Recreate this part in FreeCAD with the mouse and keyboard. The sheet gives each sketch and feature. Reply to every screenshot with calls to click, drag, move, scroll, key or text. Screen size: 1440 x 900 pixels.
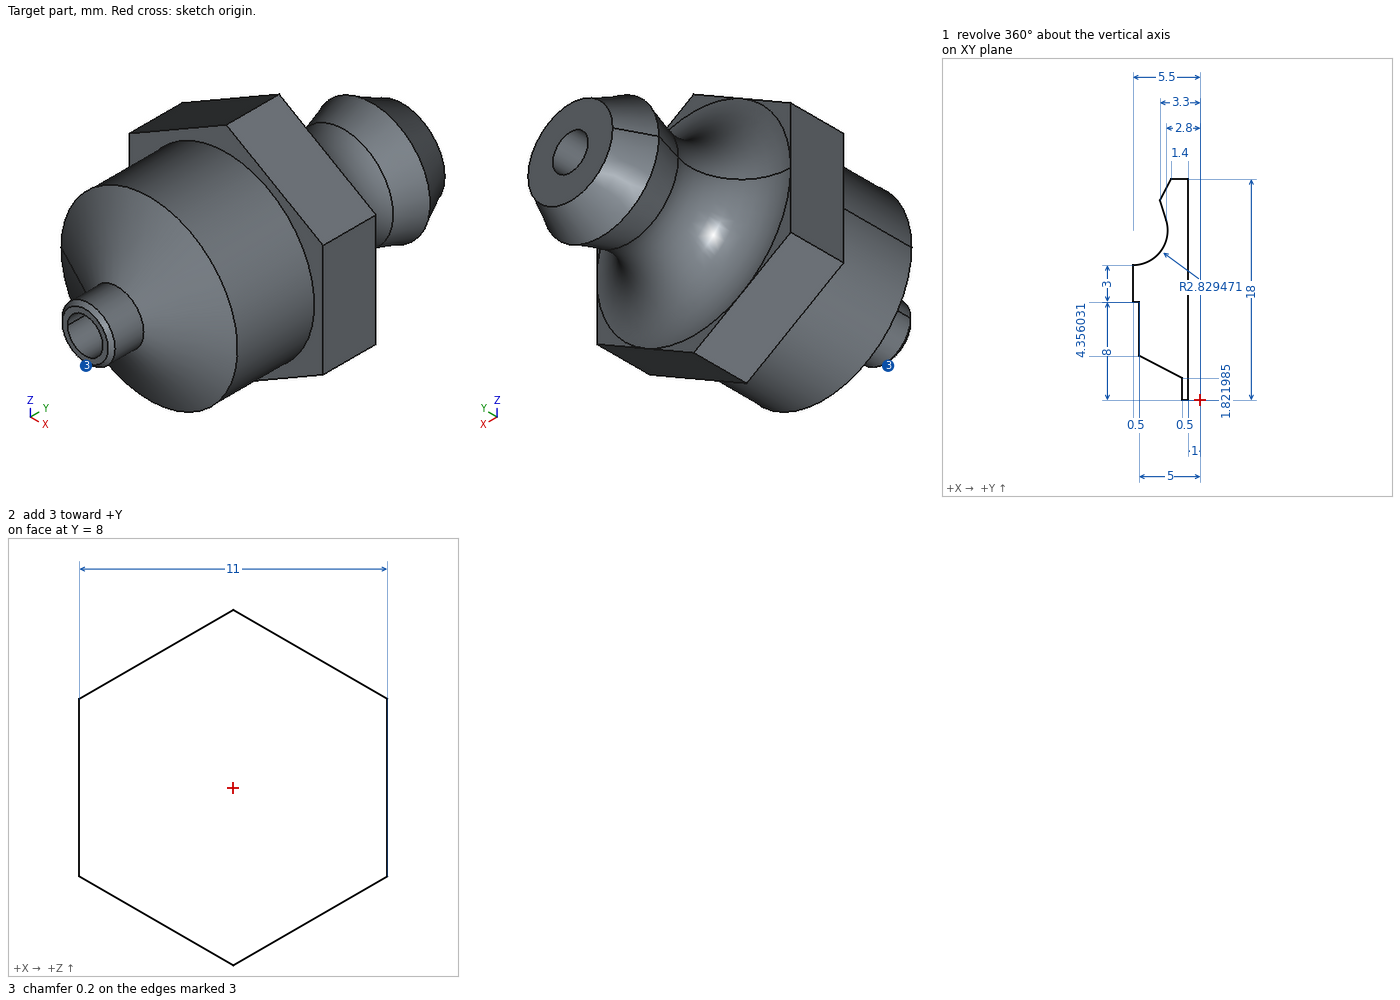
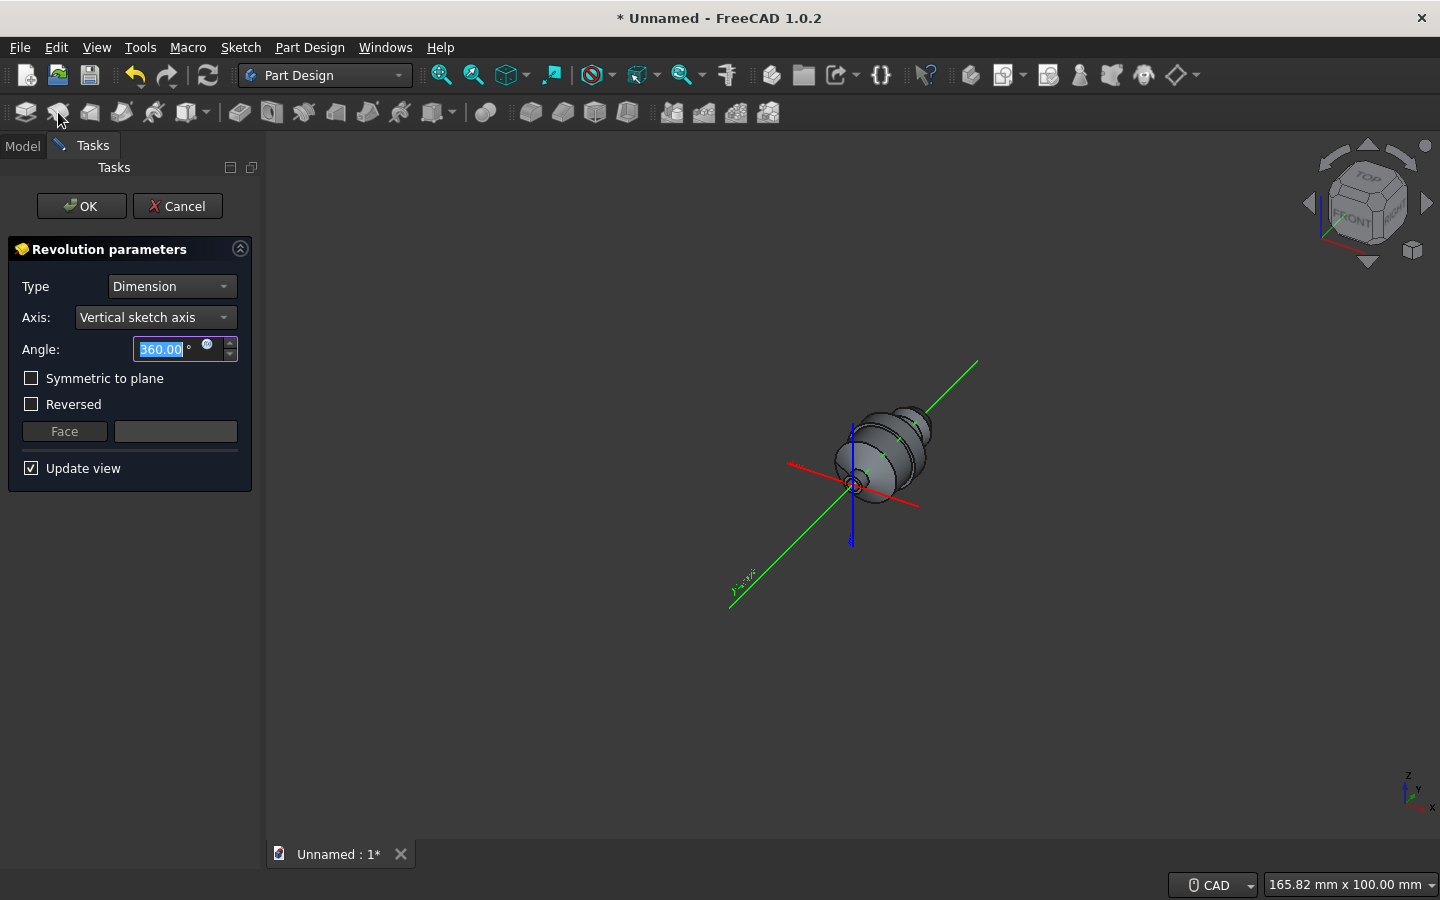
click(82, 206)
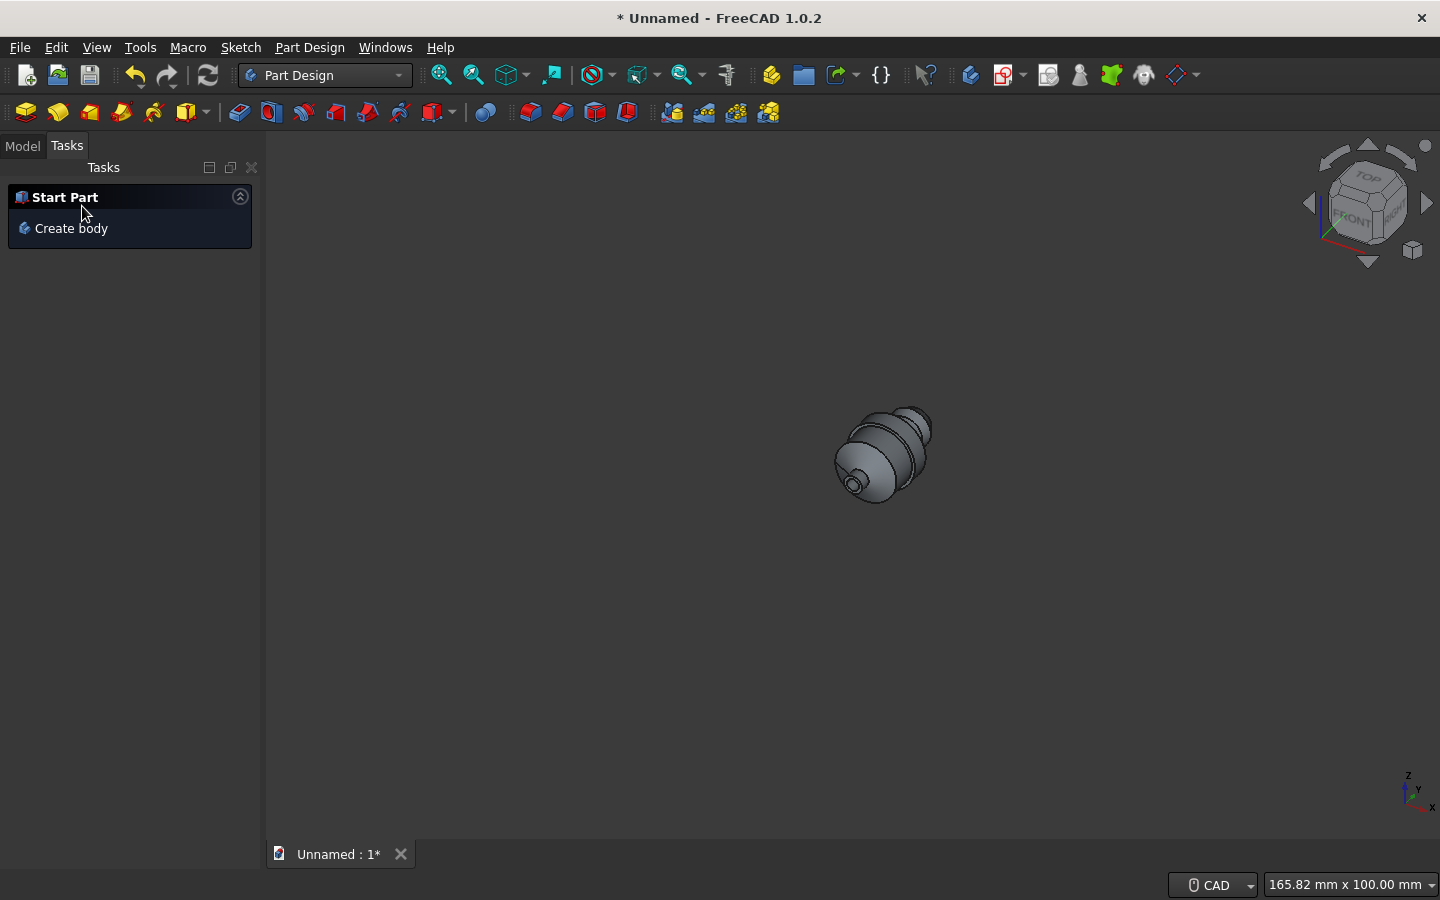
click(442, 76)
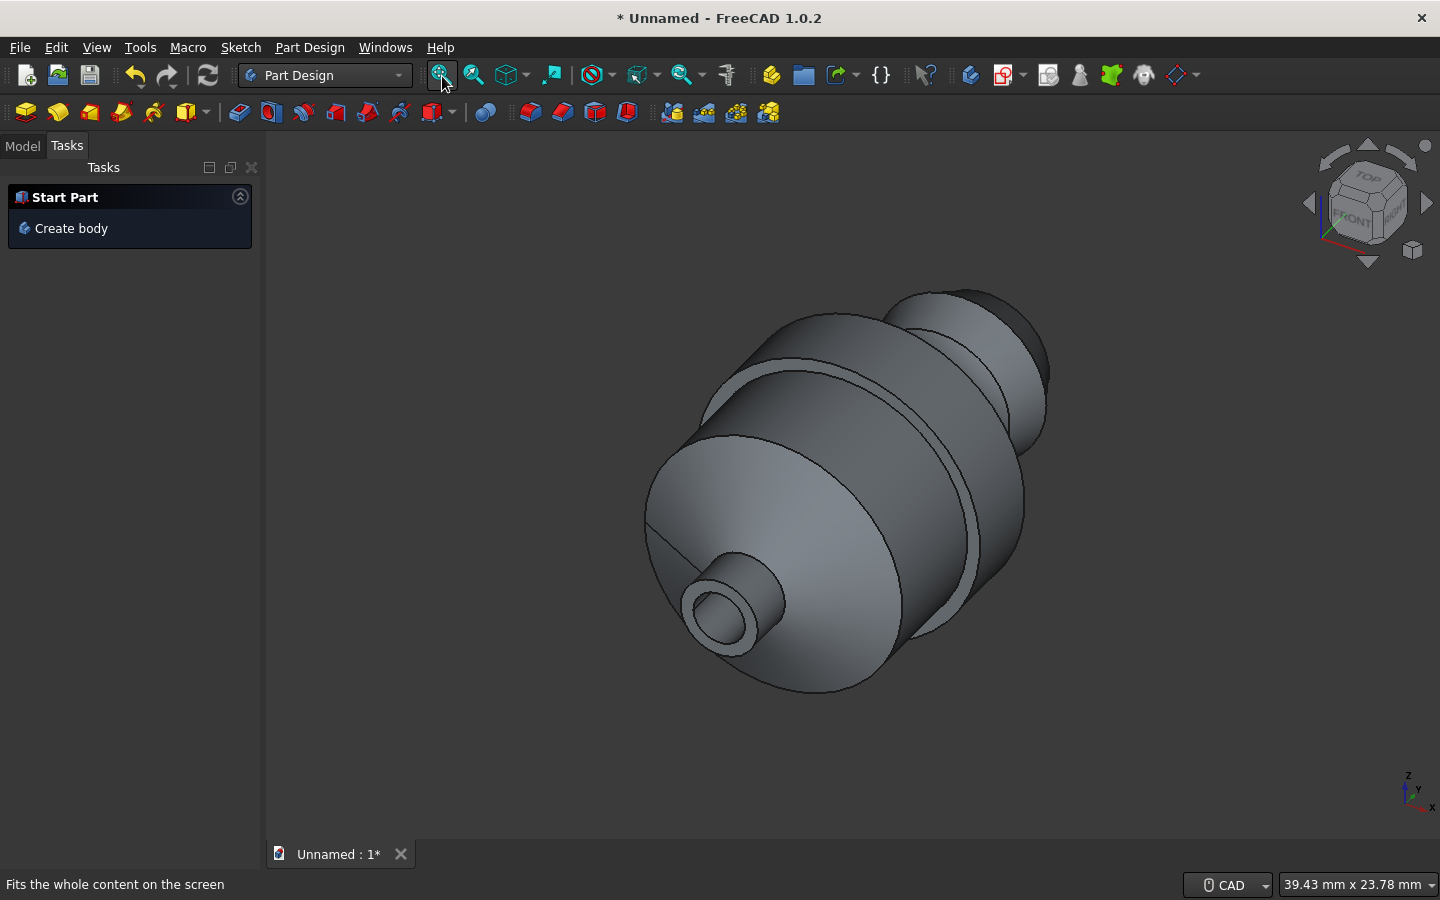
scroll(976, 542, up, 5)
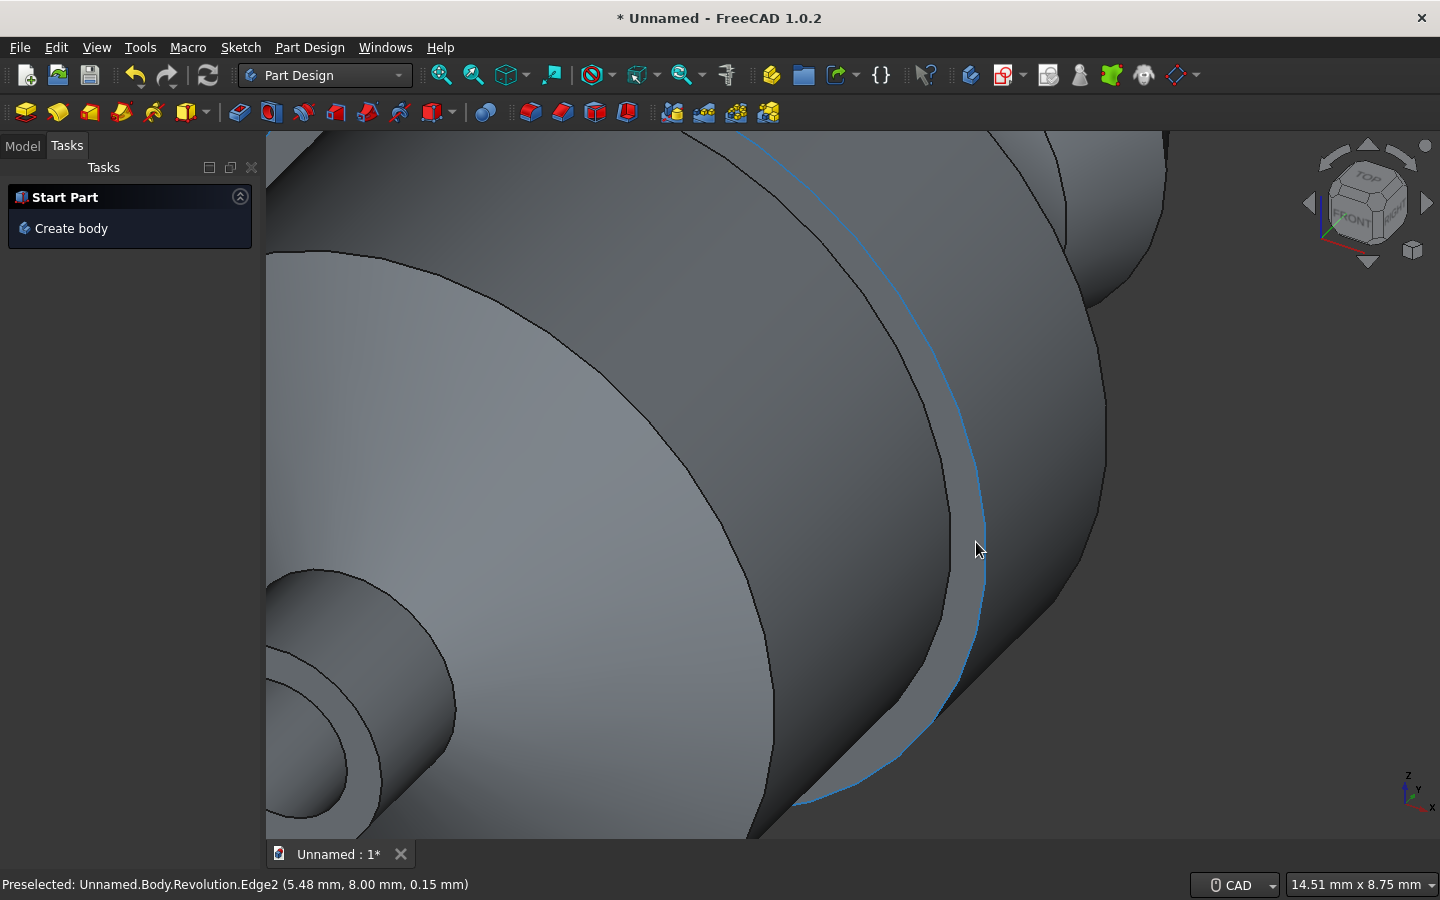
click(974, 543)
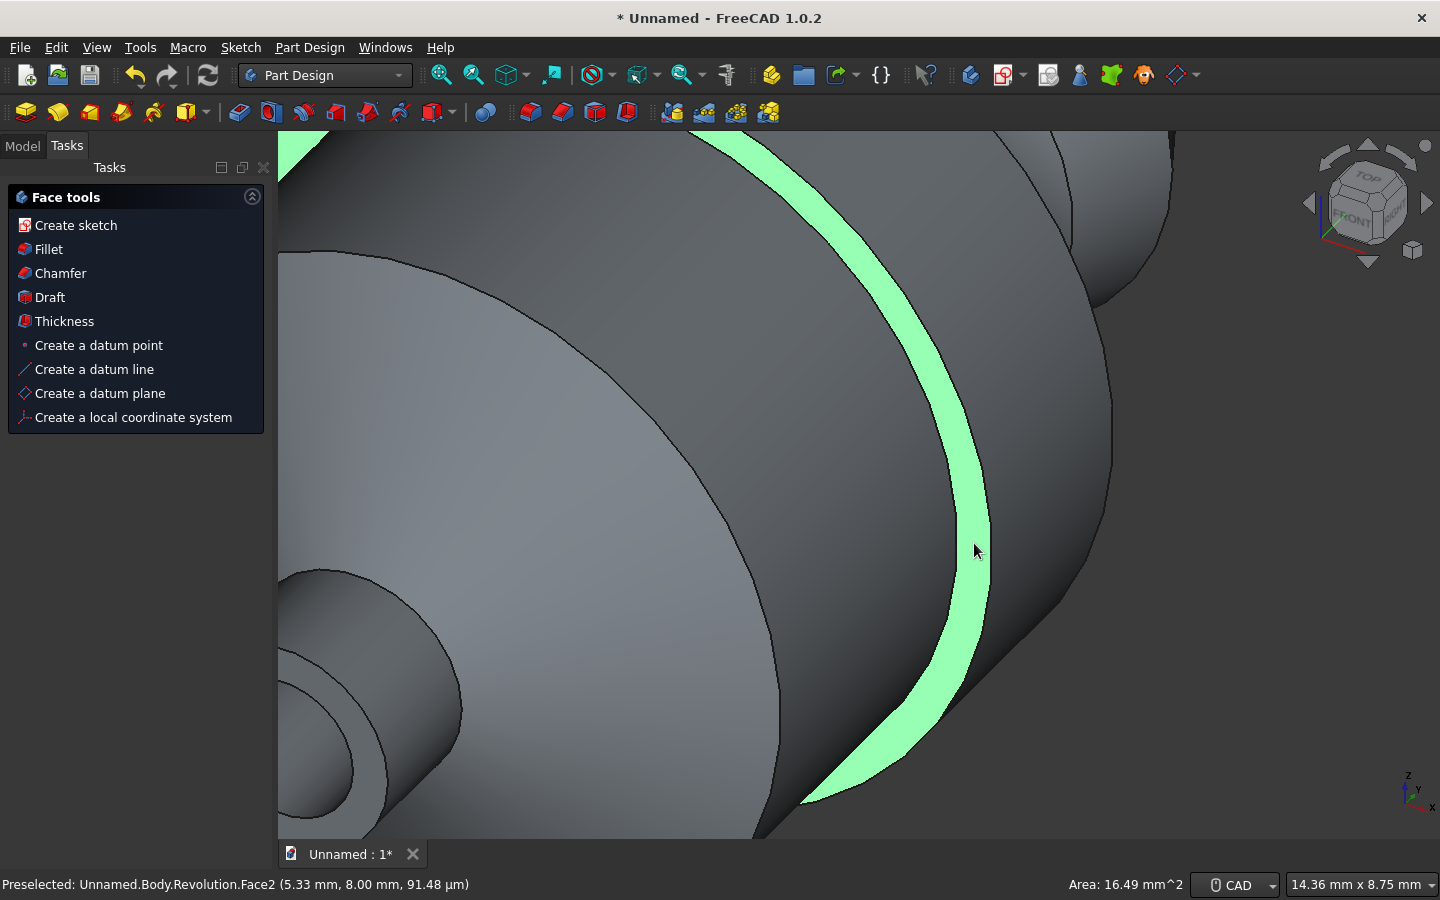
click(1004, 76)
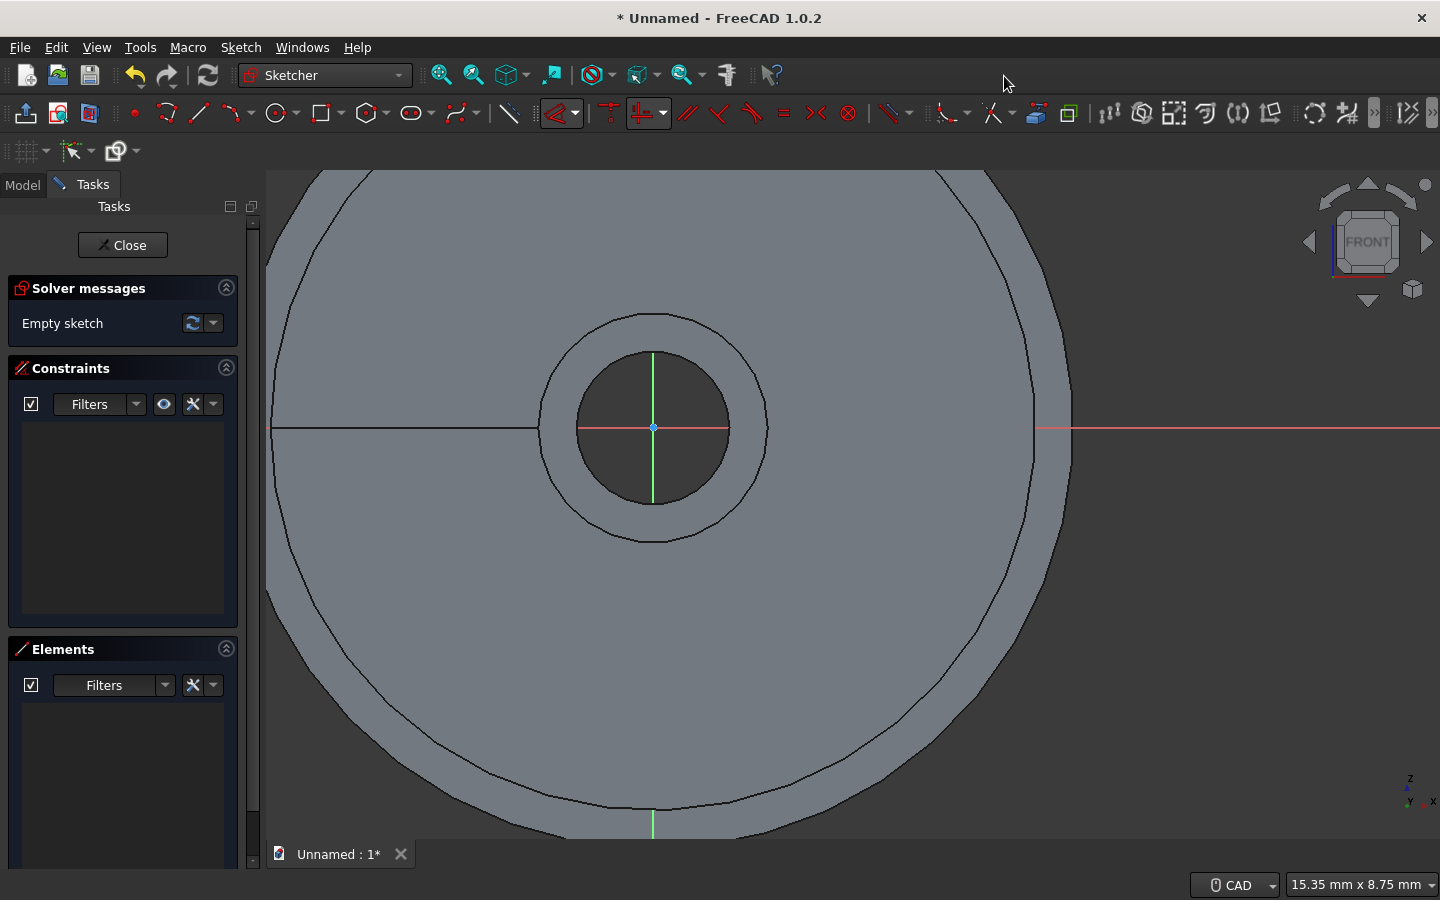
click(90, 114)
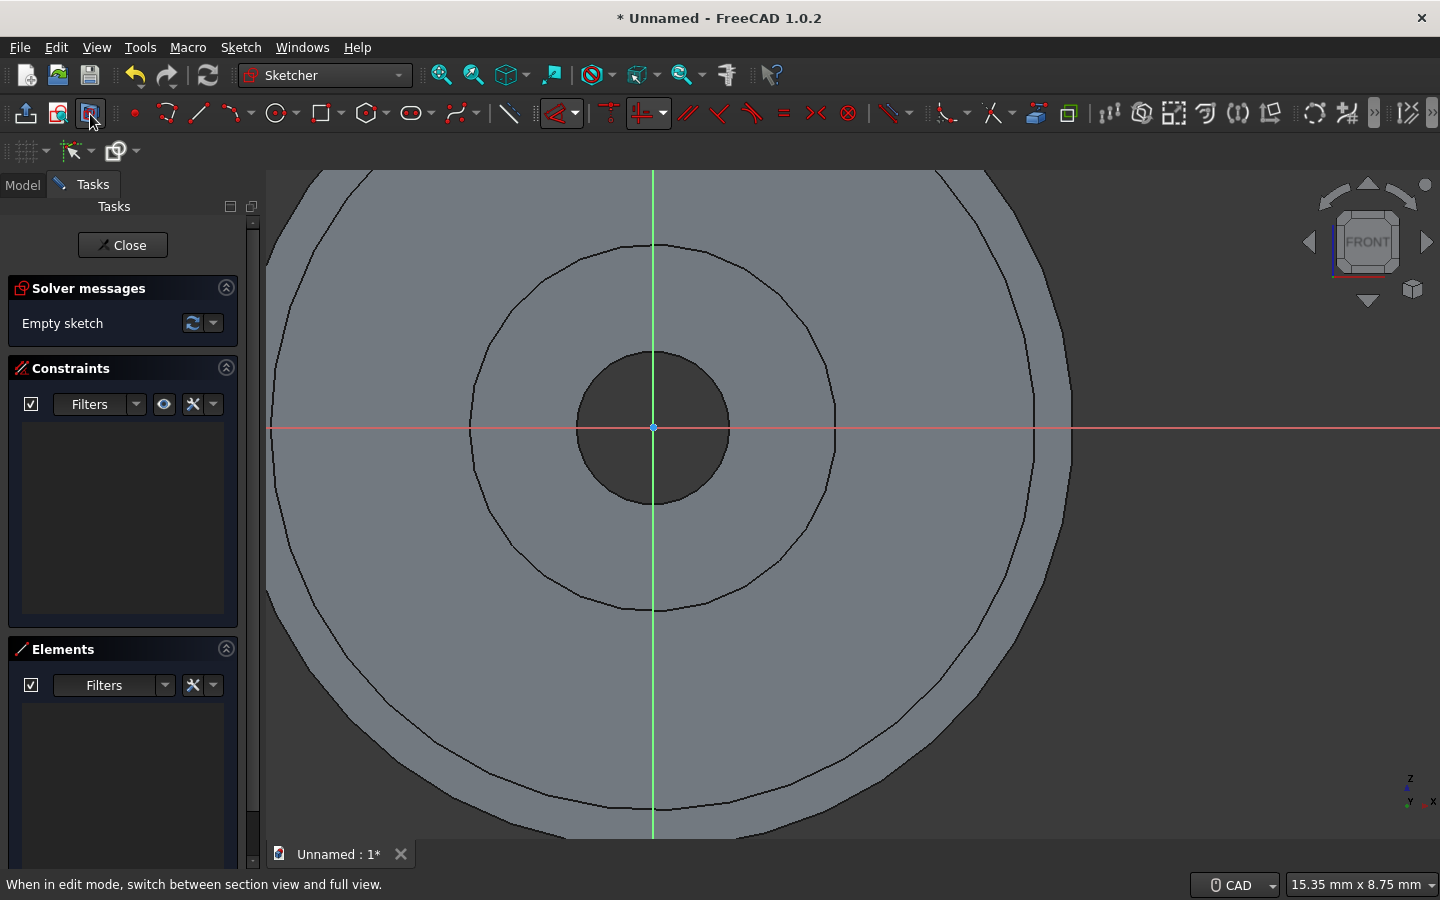
scroll(892, 567, down, 4)